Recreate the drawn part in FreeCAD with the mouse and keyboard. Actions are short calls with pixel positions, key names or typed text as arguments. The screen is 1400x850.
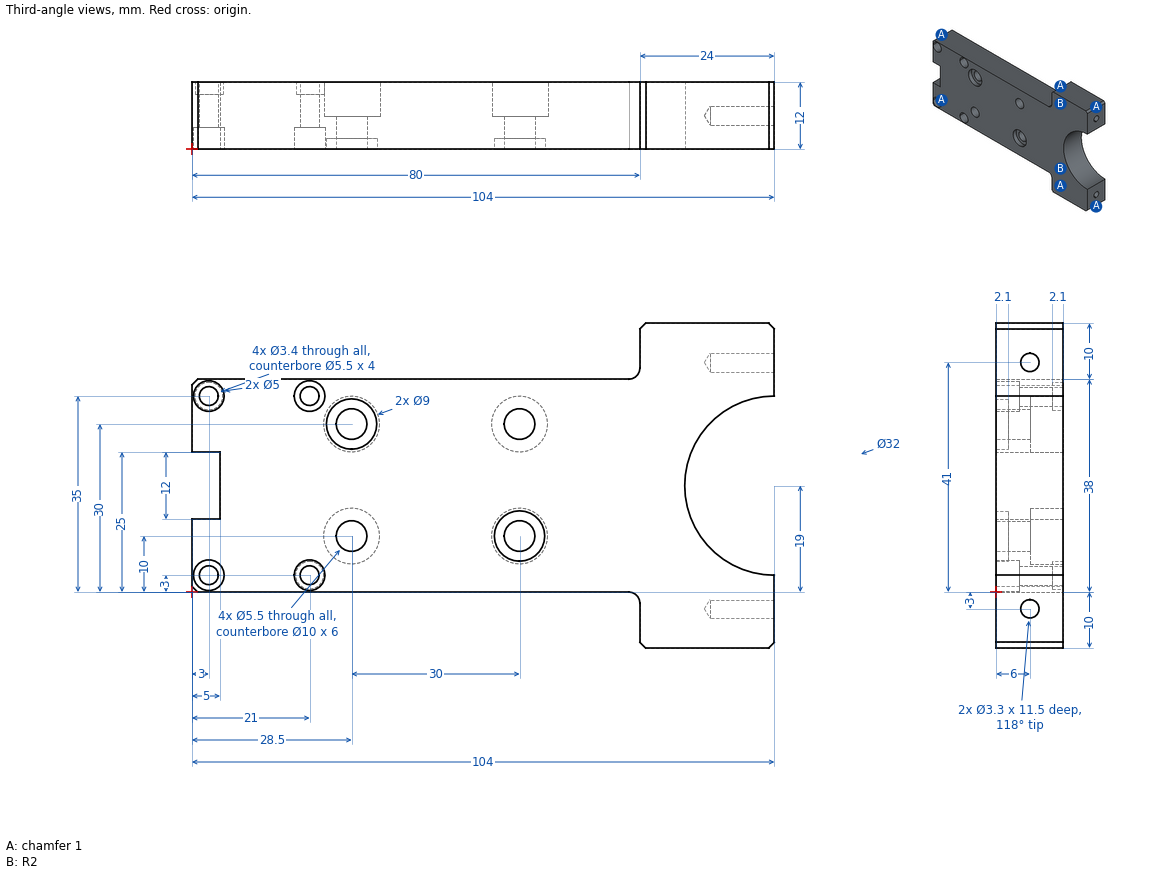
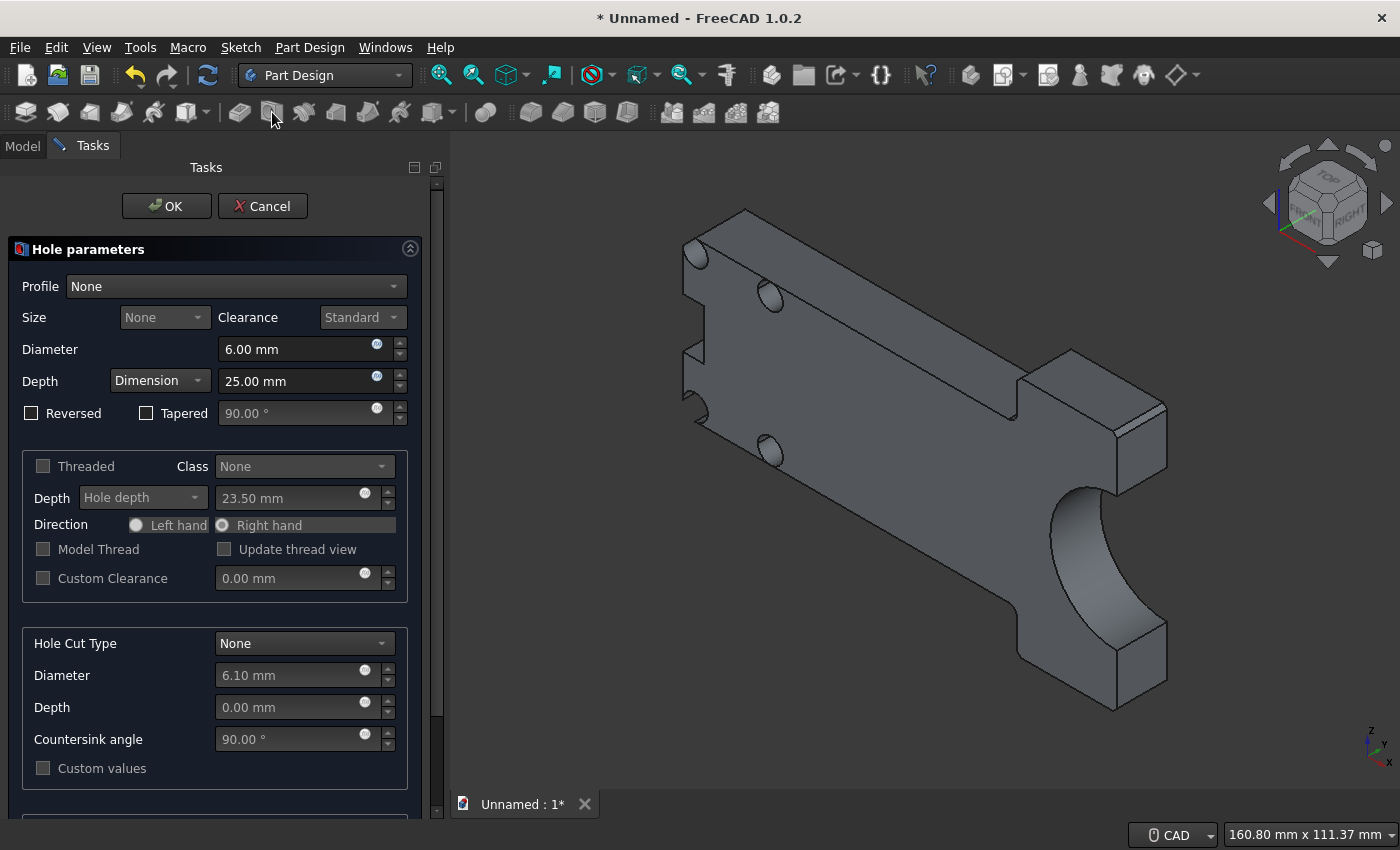
triple_click(305, 349)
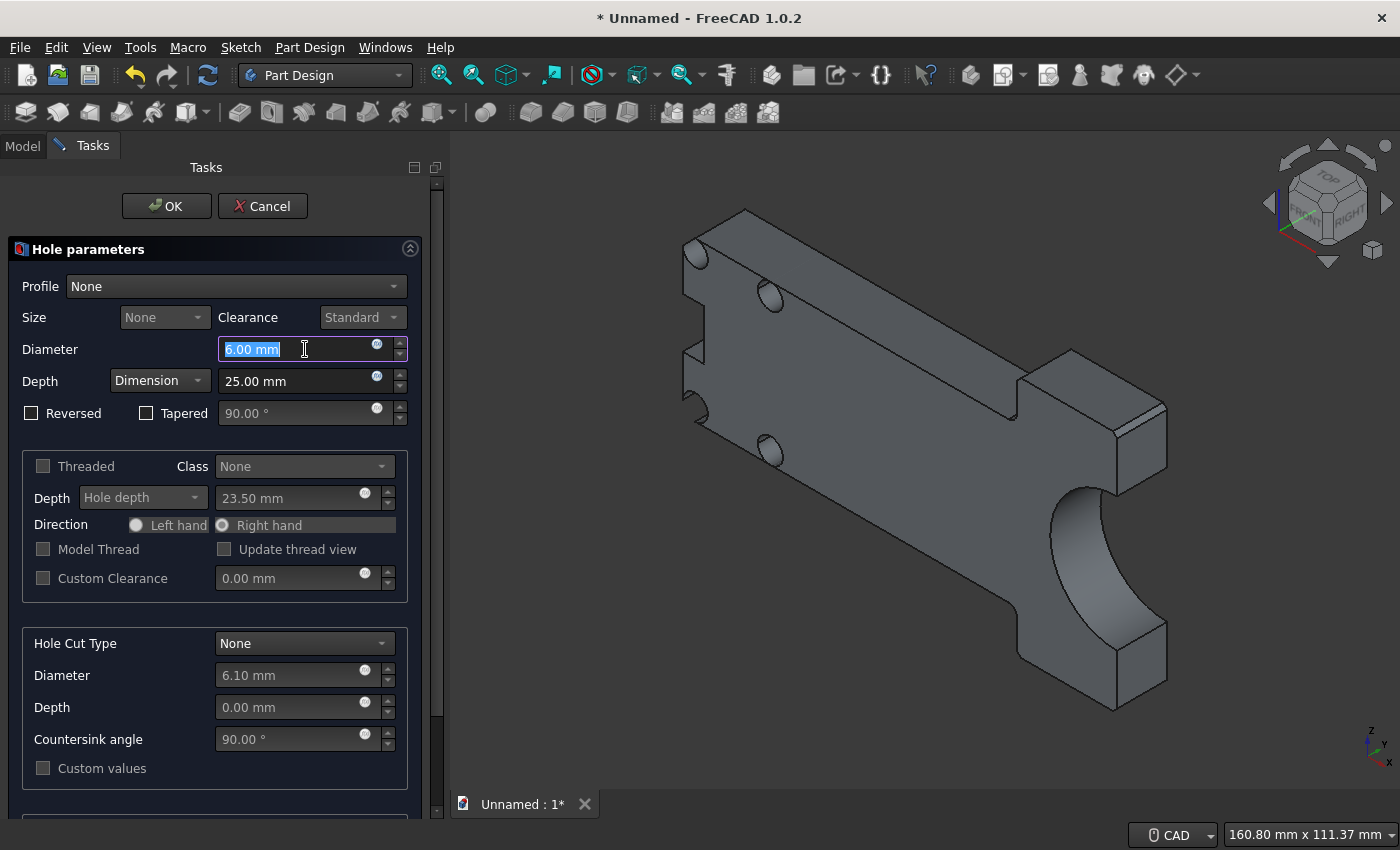
text(3.4)
key(Tab)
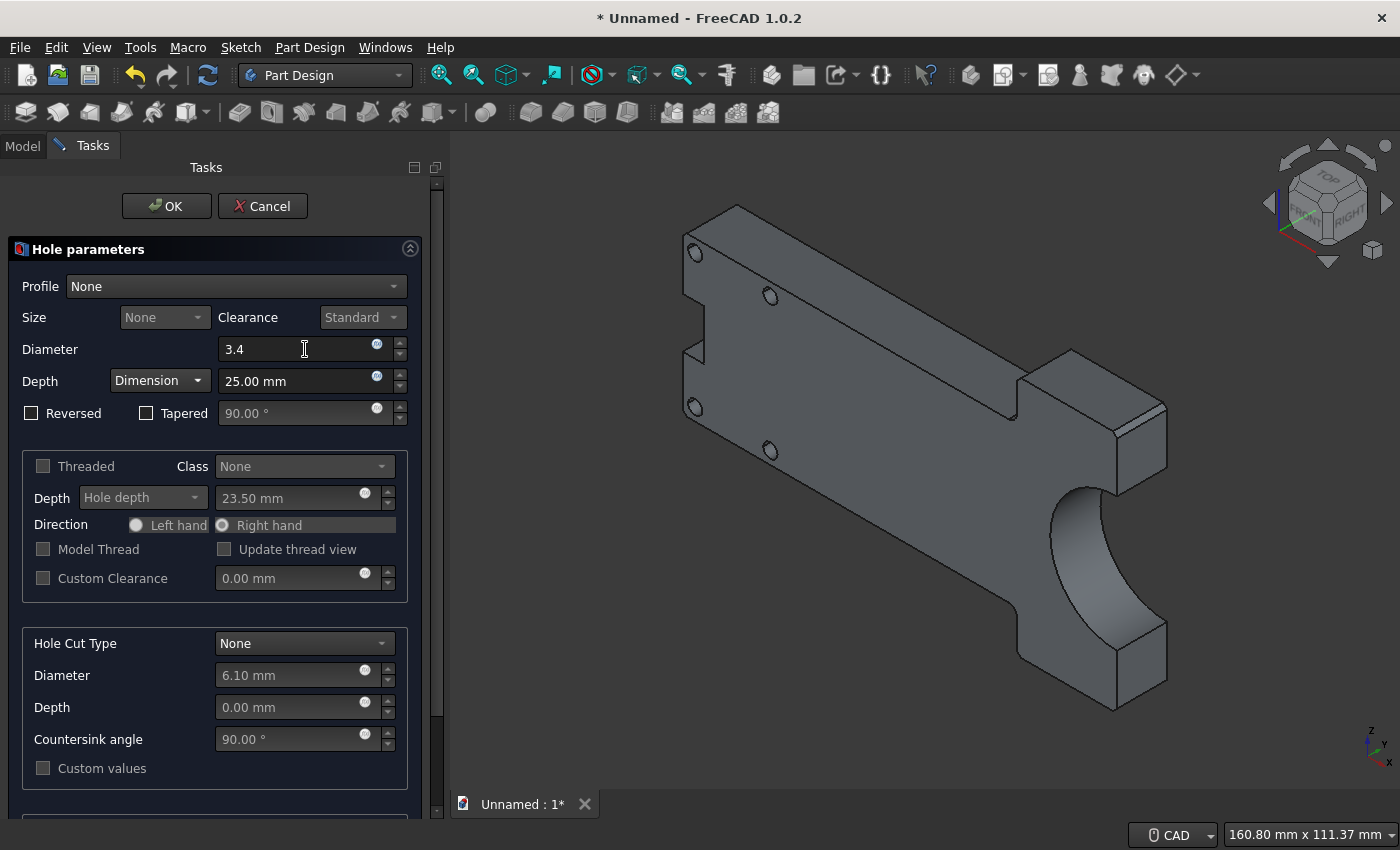
click(161, 380)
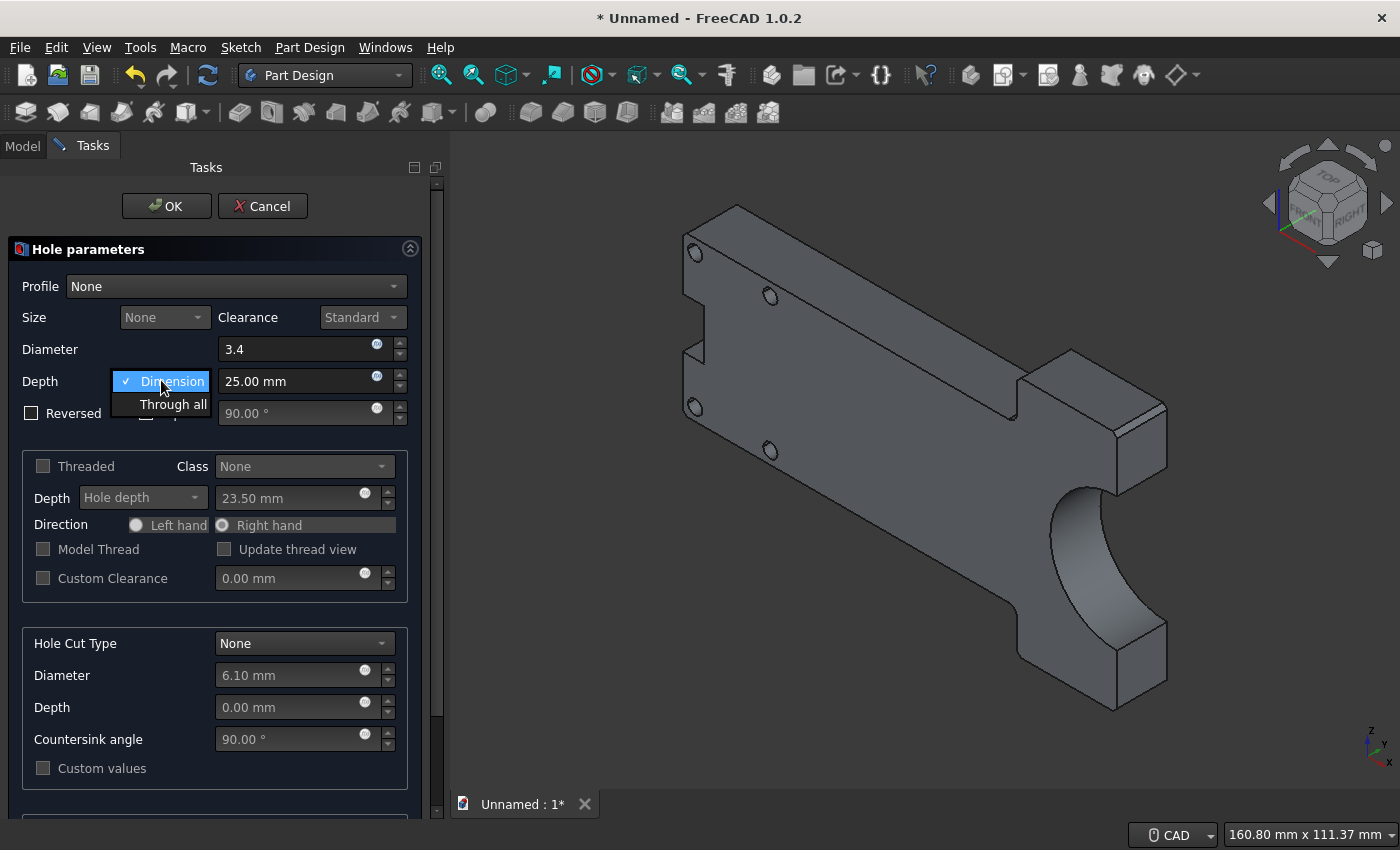
click(160, 404)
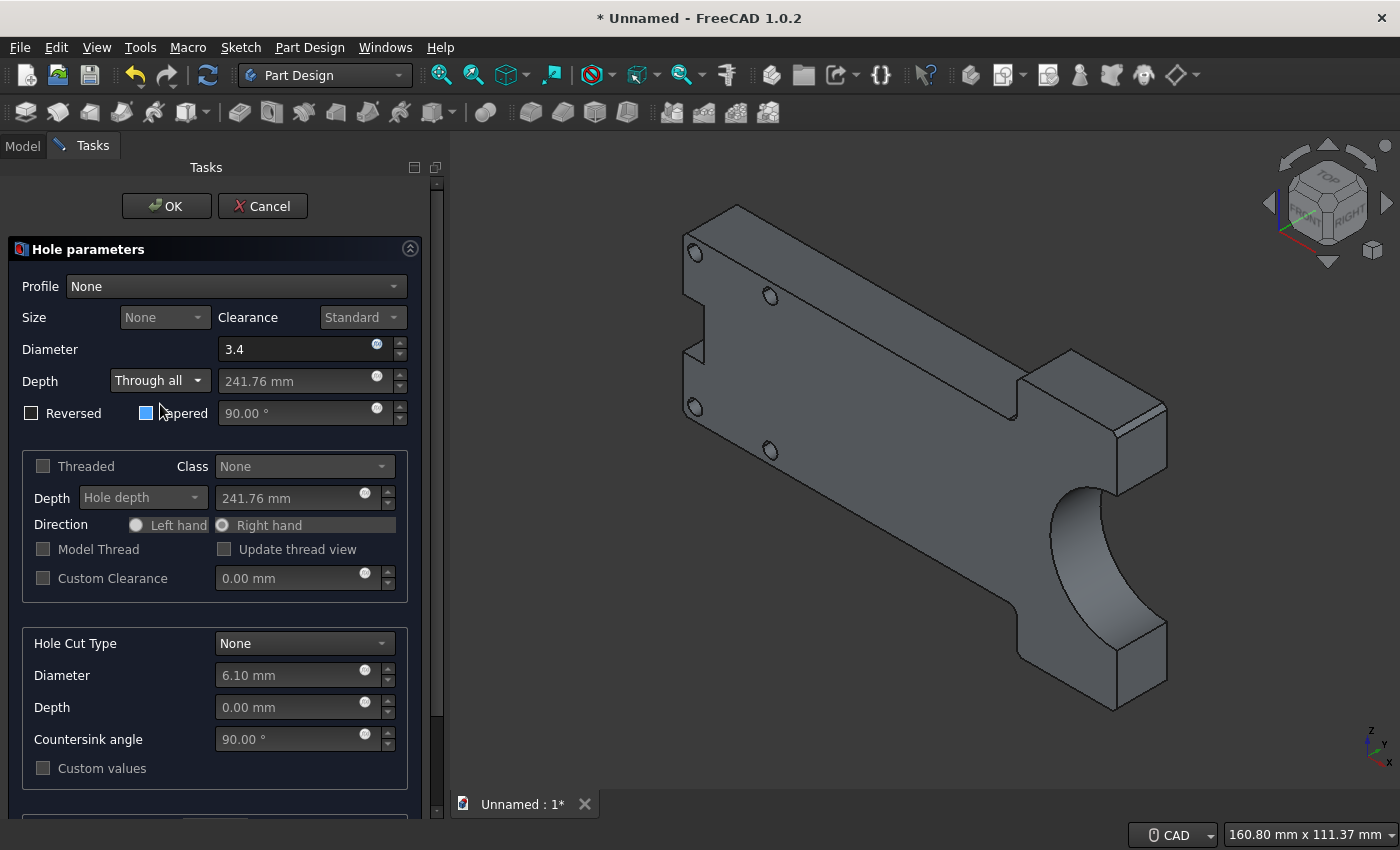
click(306, 644)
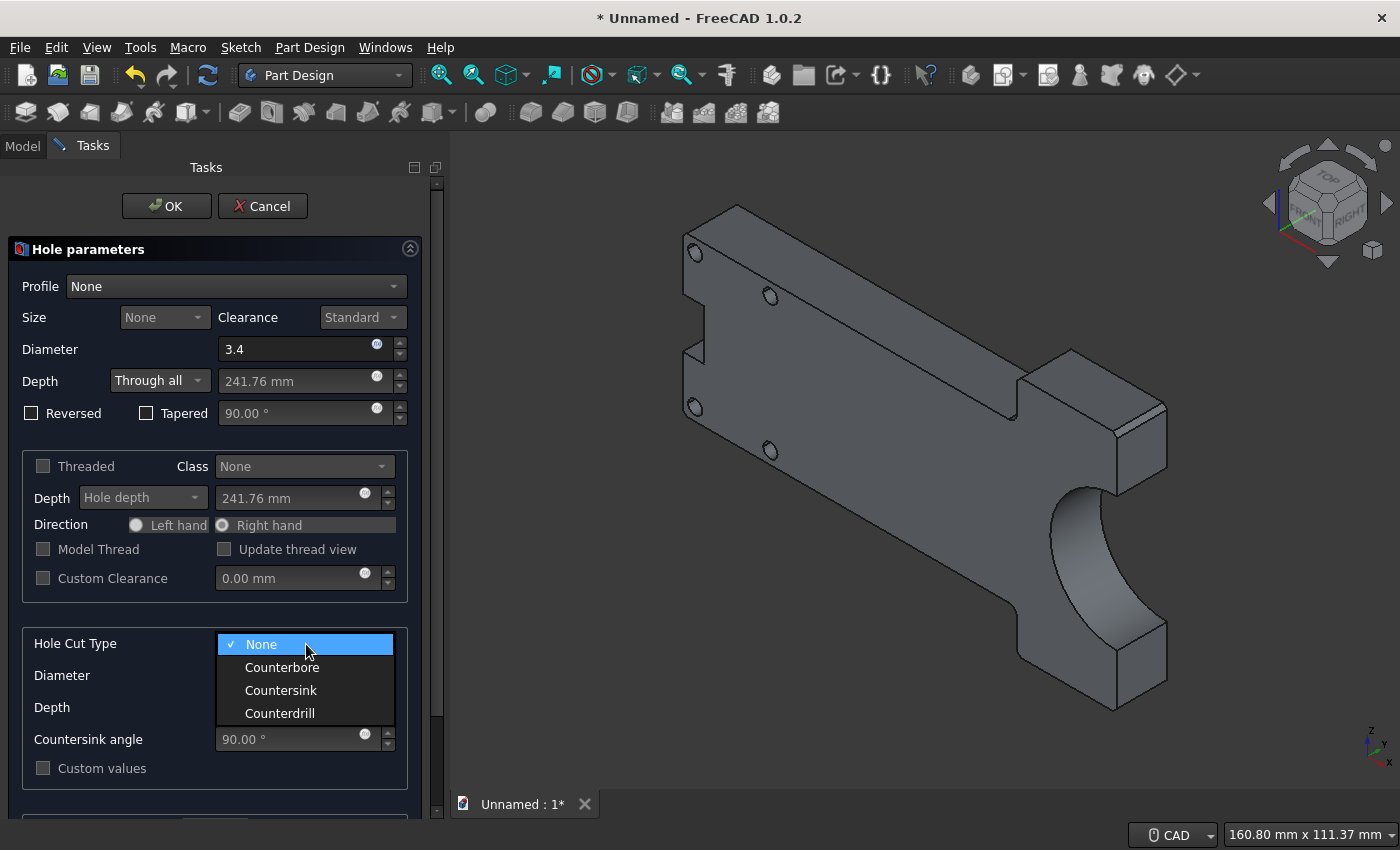
click(304, 668)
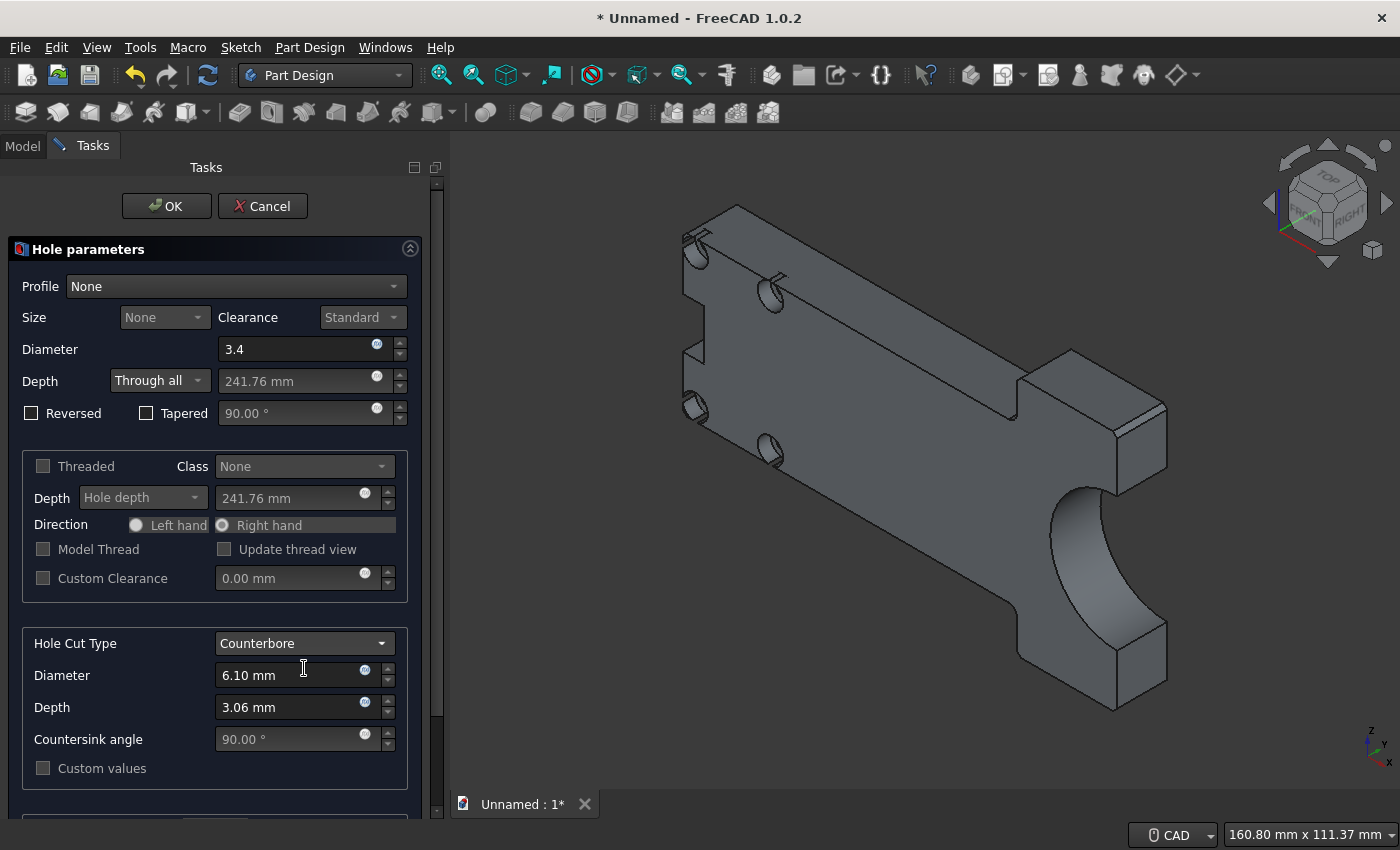
triple_click(298, 675)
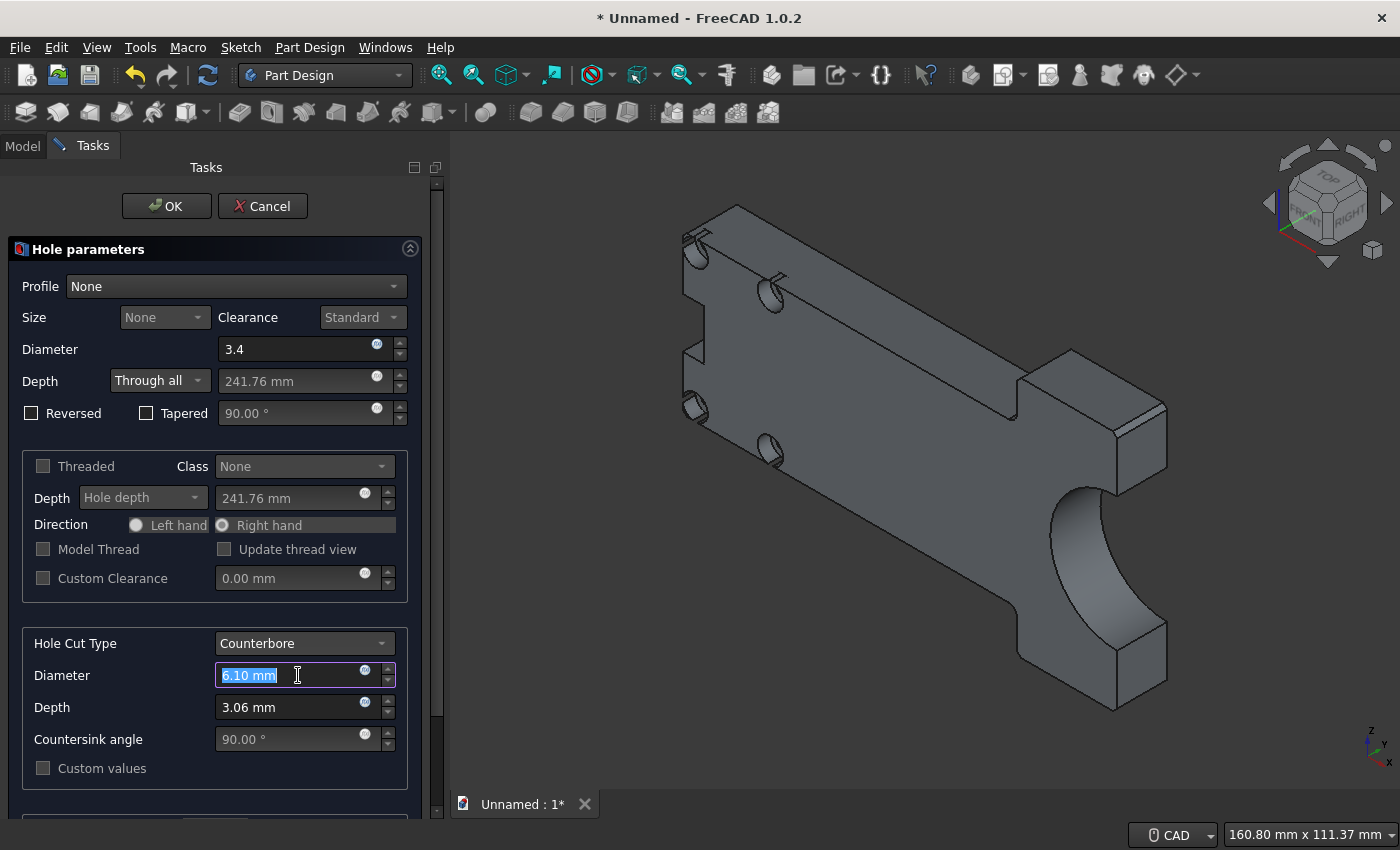
text(5.5)
key(Tab)